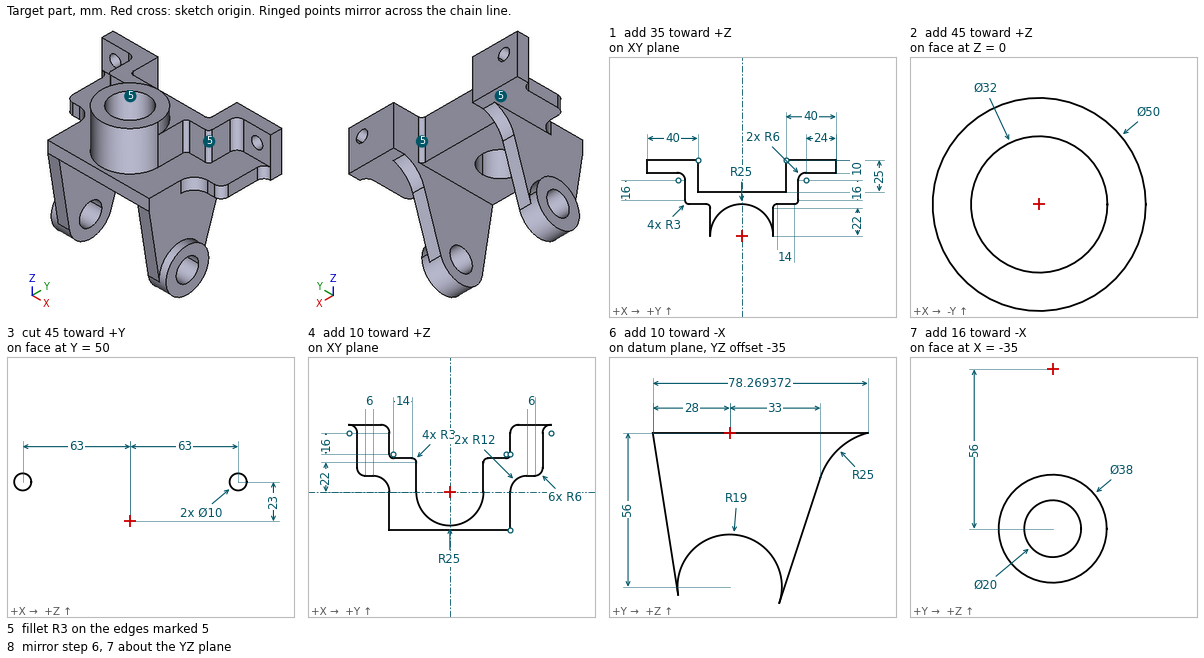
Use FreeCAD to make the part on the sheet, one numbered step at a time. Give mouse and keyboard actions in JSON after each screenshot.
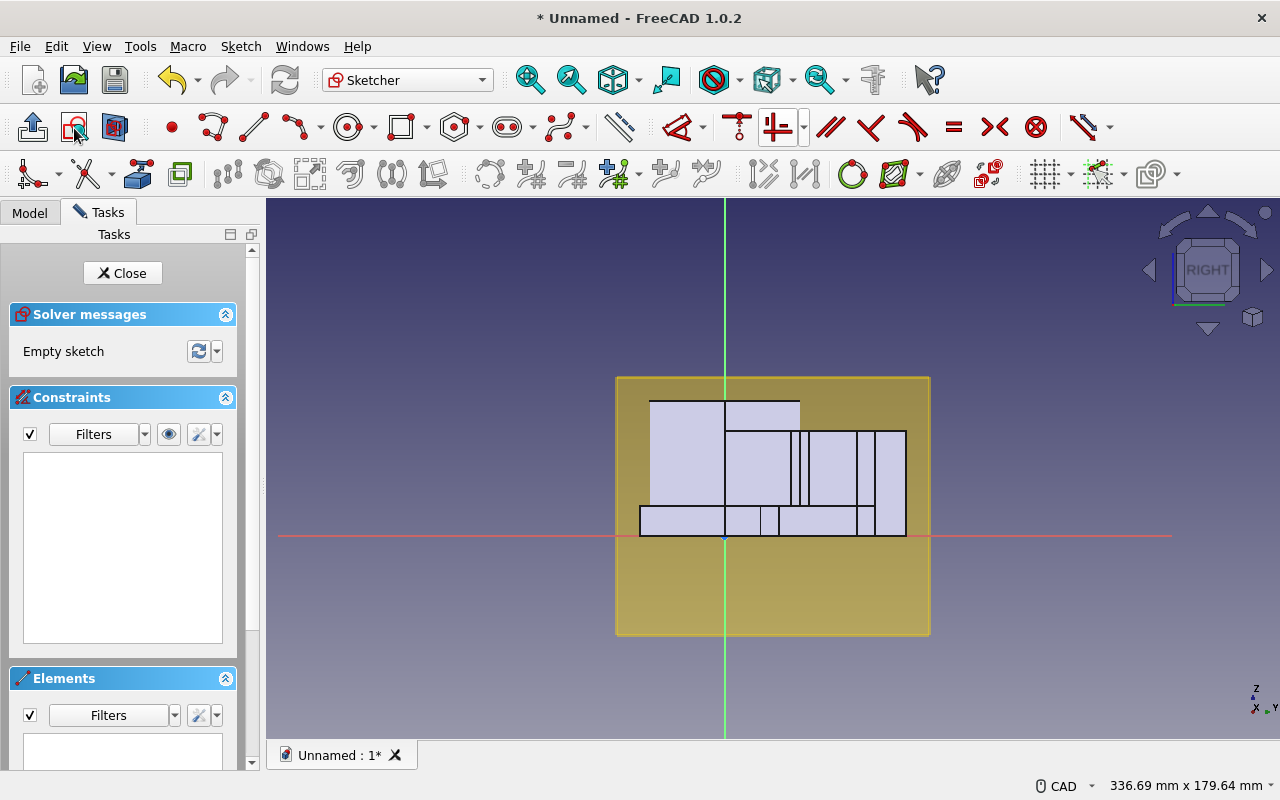
{"action": "left_click", "coordinate": [115, 128]}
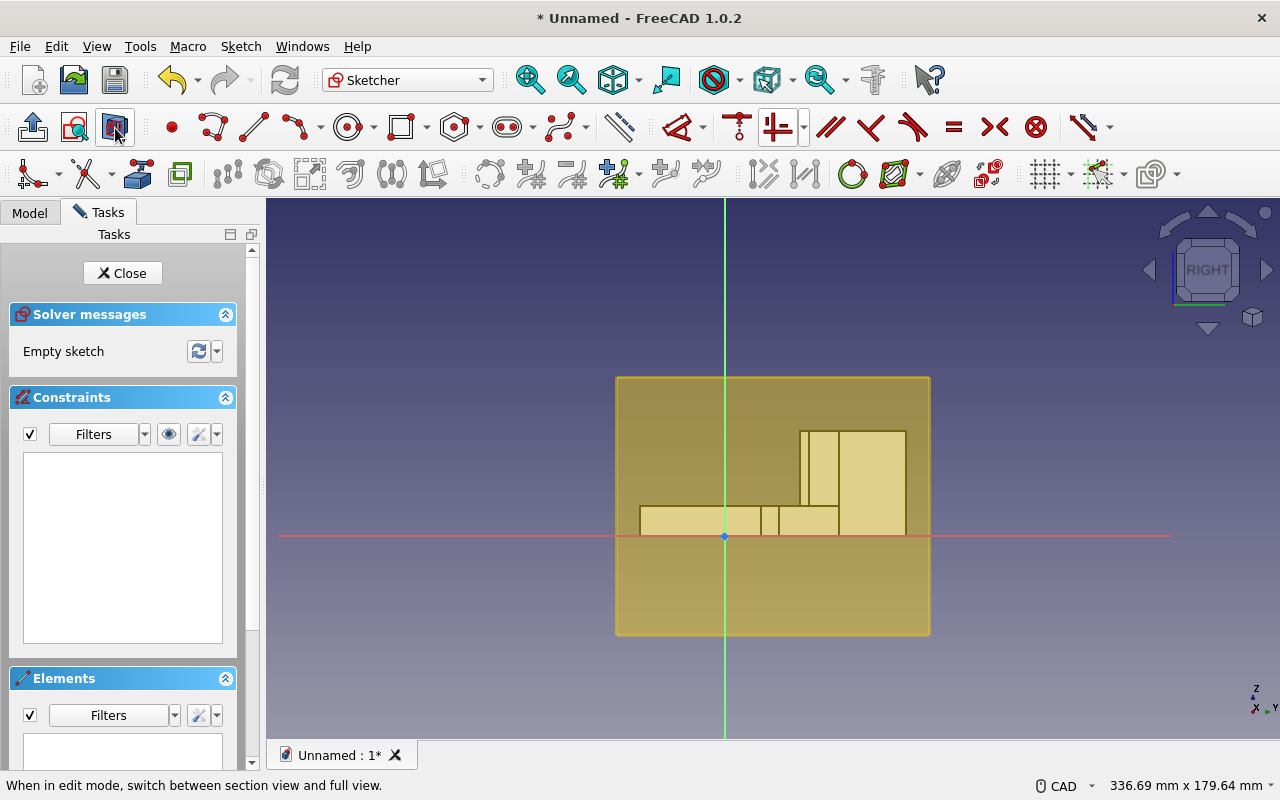
{"action": "scroll", "coordinate": [704, 468], "scroll_direction": "down", "scroll_amount": 5}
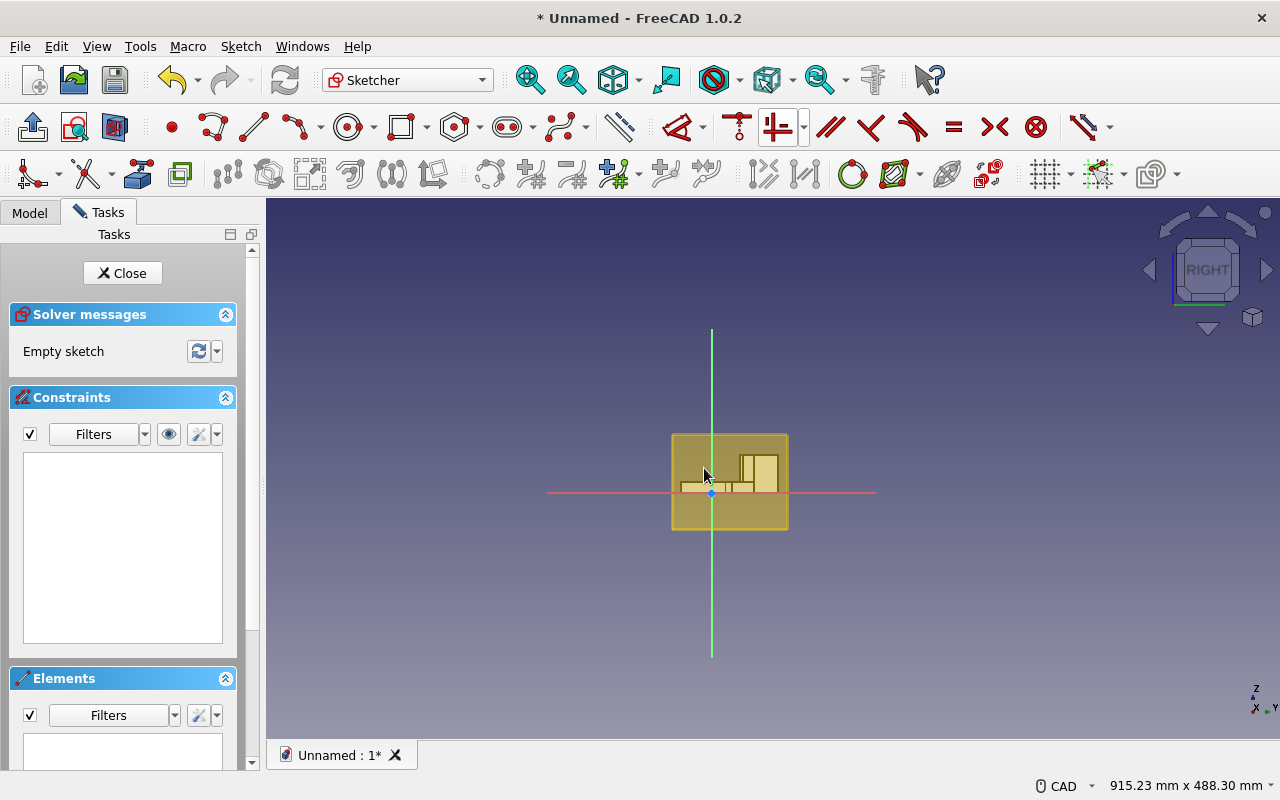
{"action": "scroll", "coordinate": [729, 543], "scroll_direction": "up", "scroll_amount": 8}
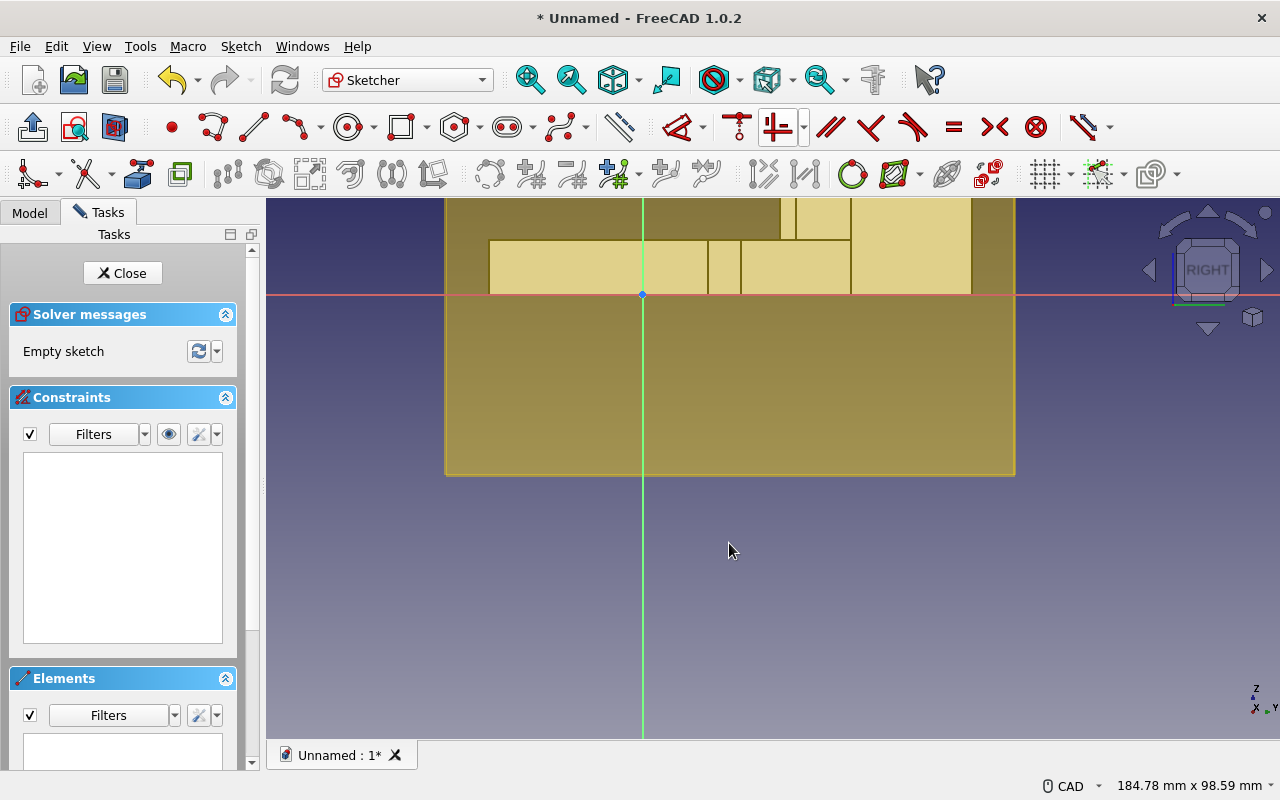
{"action": "left_click", "coordinate": [254, 128]}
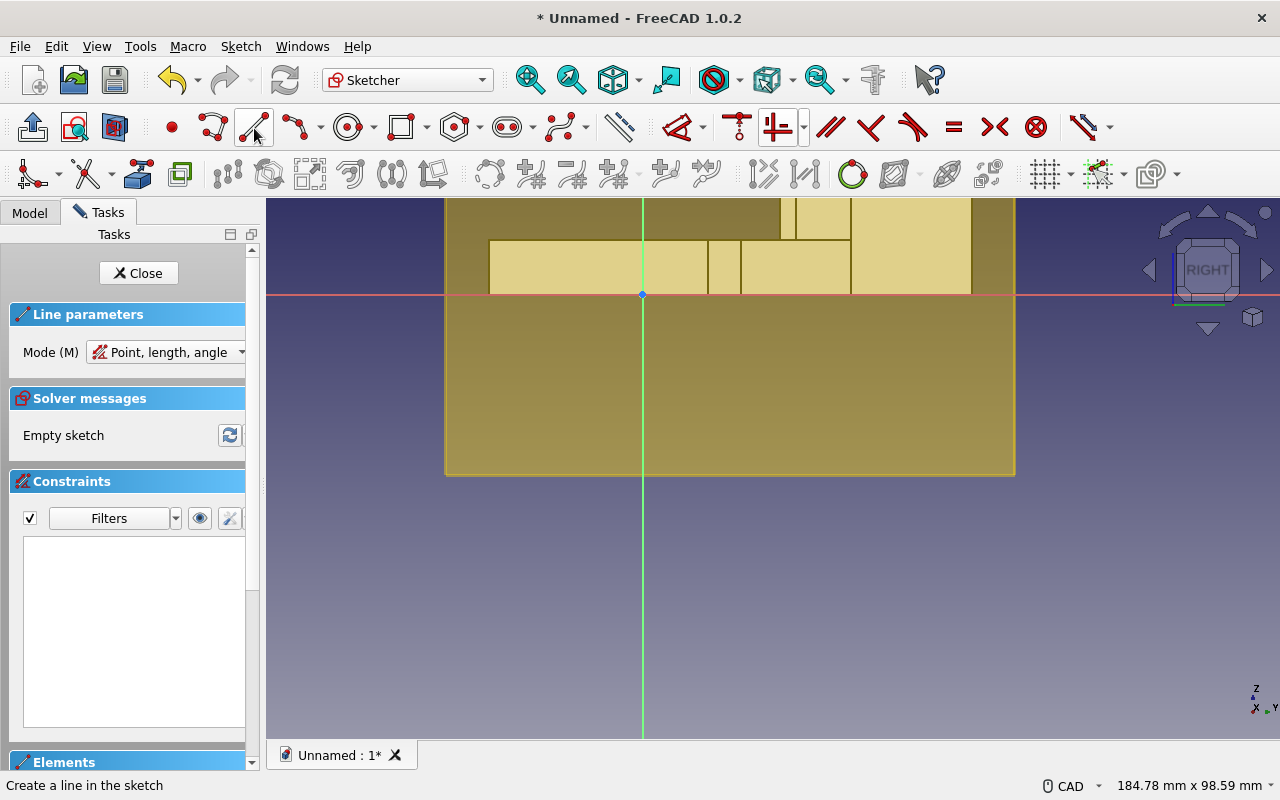
{"action": "left_click", "coordinate": [742, 635]}
{"action": "left_click", "coordinate": [824, 385]}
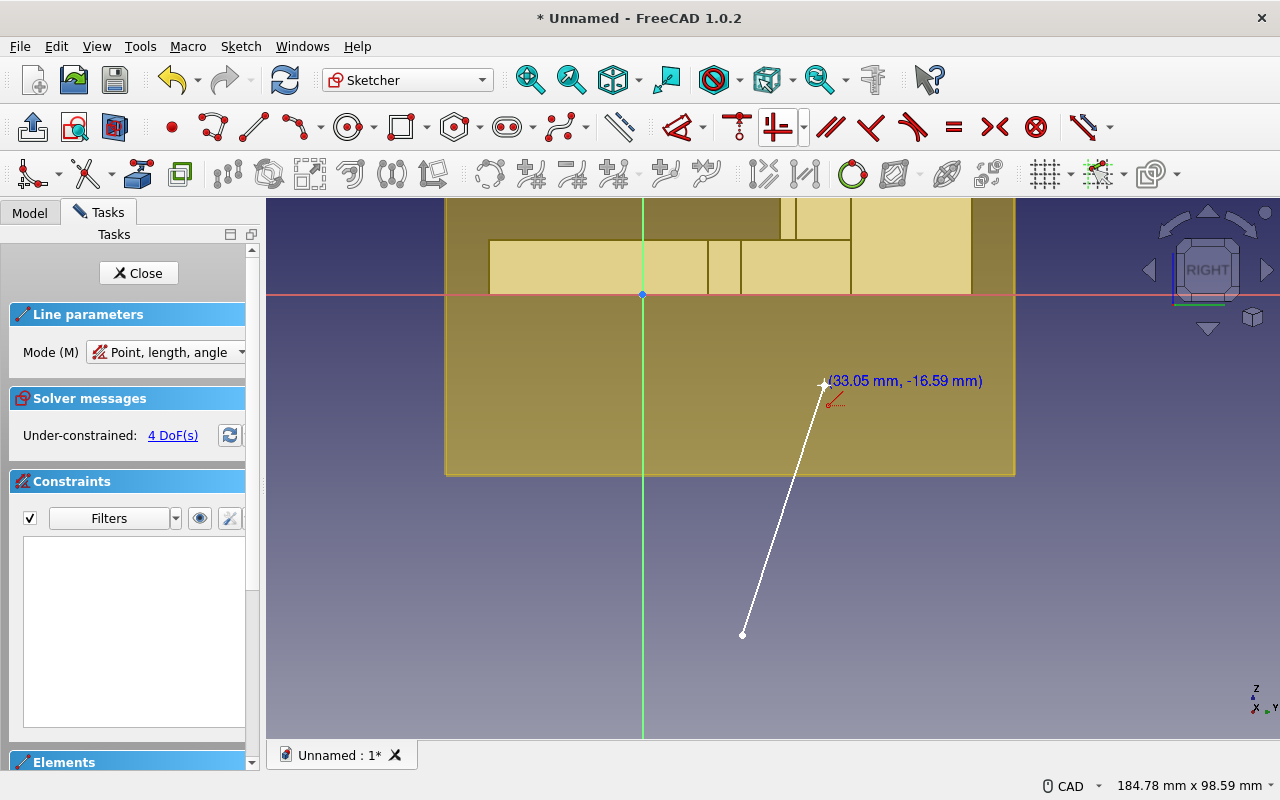
{"action": "left_click", "coordinate": [213, 128]}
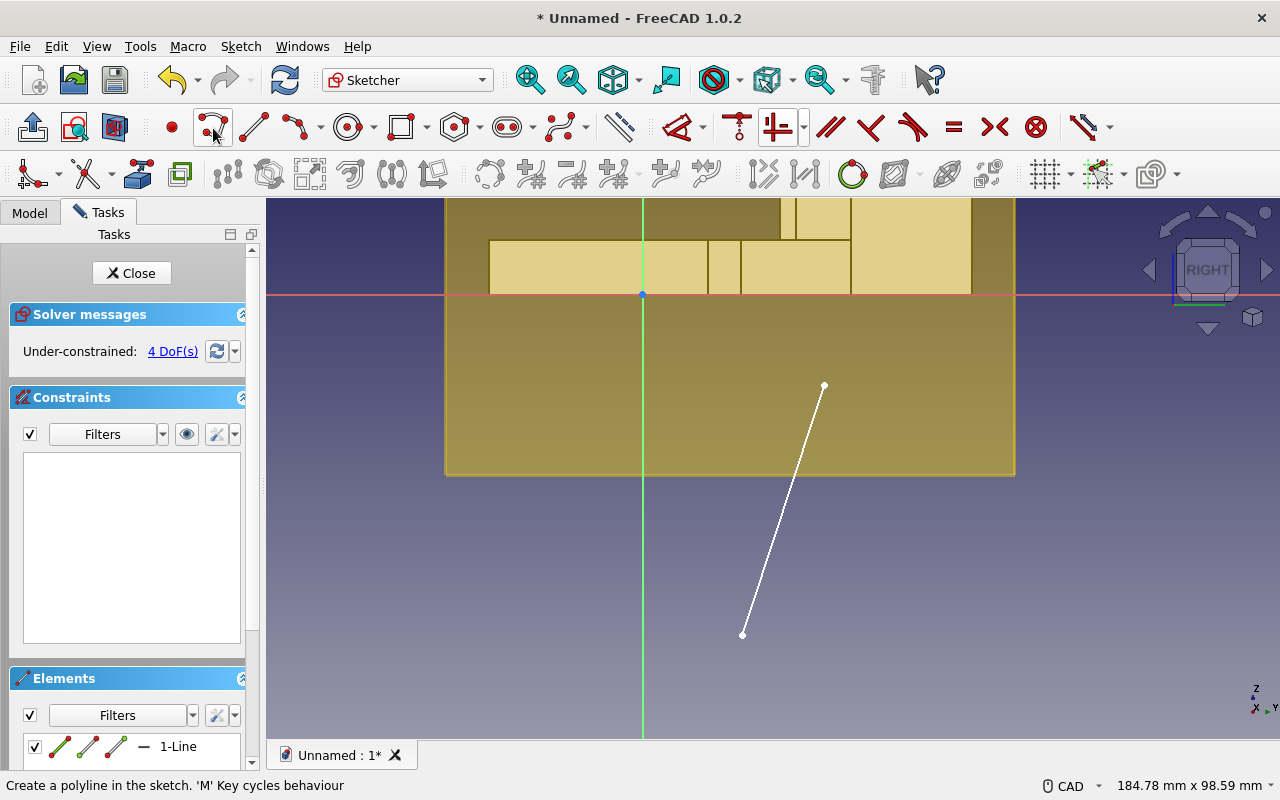
{"action": "left_click", "coordinate": [919, 295]}
{"action": "left_click", "coordinate": [489, 304]}
{"action": "left_click", "coordinate": [540, 618]}
{"action": "right_click", "coordinate": [540, 618]}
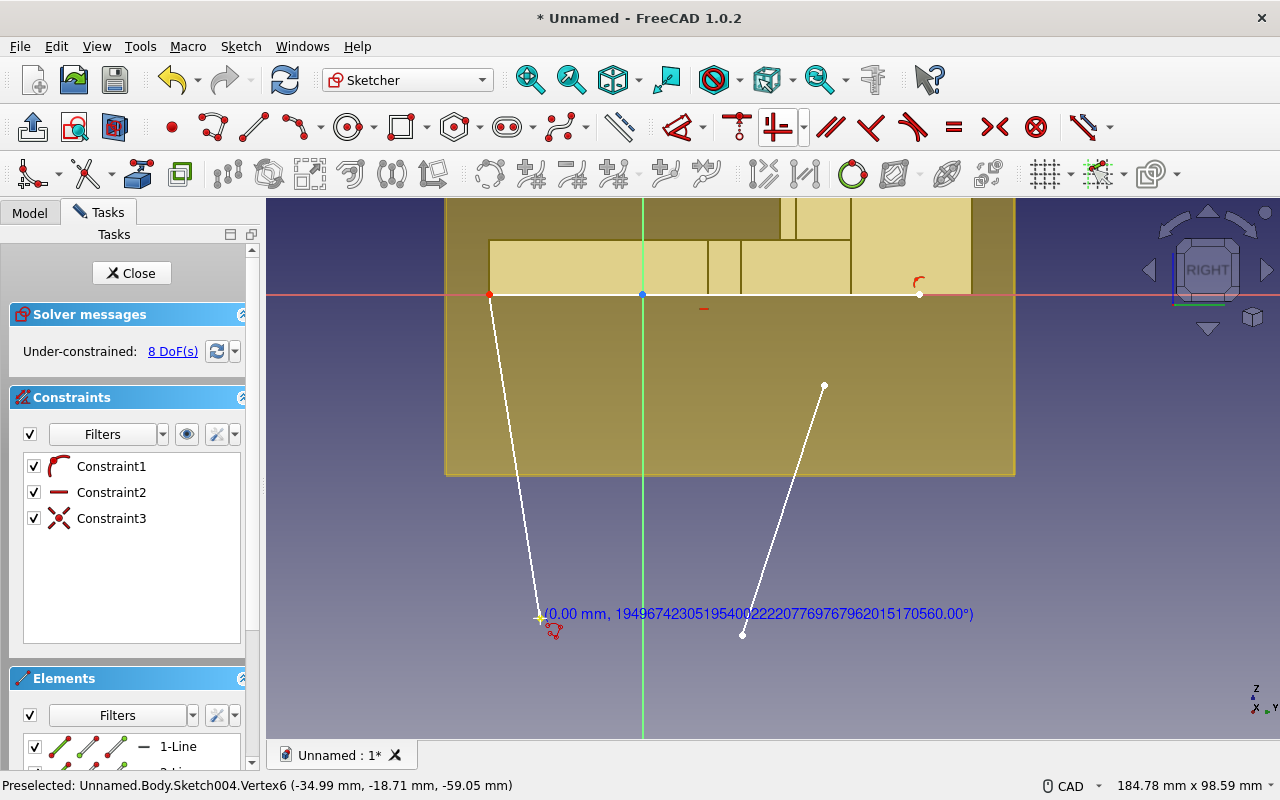
{"action": "left_click", "coordinate": [294, 128]}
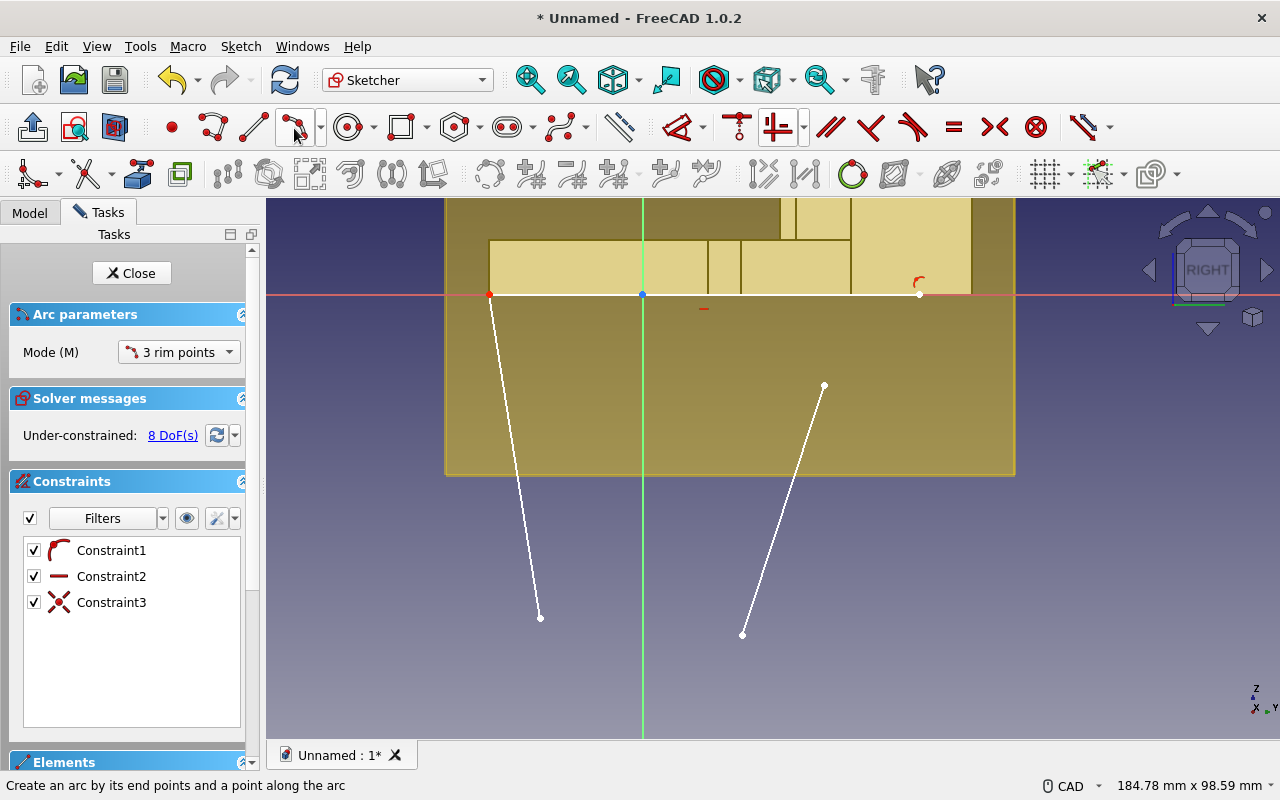
{"action": "left_click", "coordinate": [824, 386]}
{"action": "left_click", "coordinate": [919, 295]}
{"action": "left_click", "coordinate": [860, 328]}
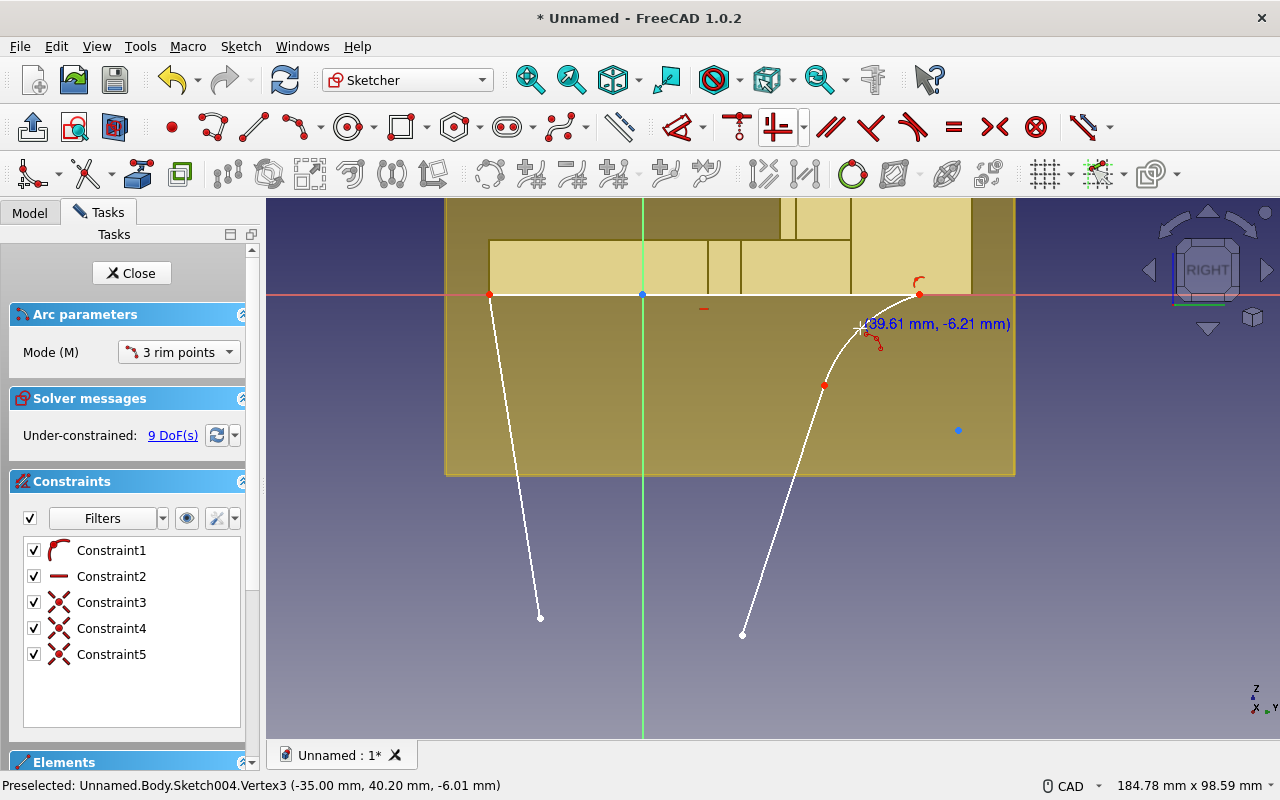
{"action": "left_click", "coordinate": [540, 619]}
{"action": "left_click", "coordinate": [742, 636]}
{"action": "left_click", "coordinate": [687, 508]}
{"action": "key", "text": "Escape"}